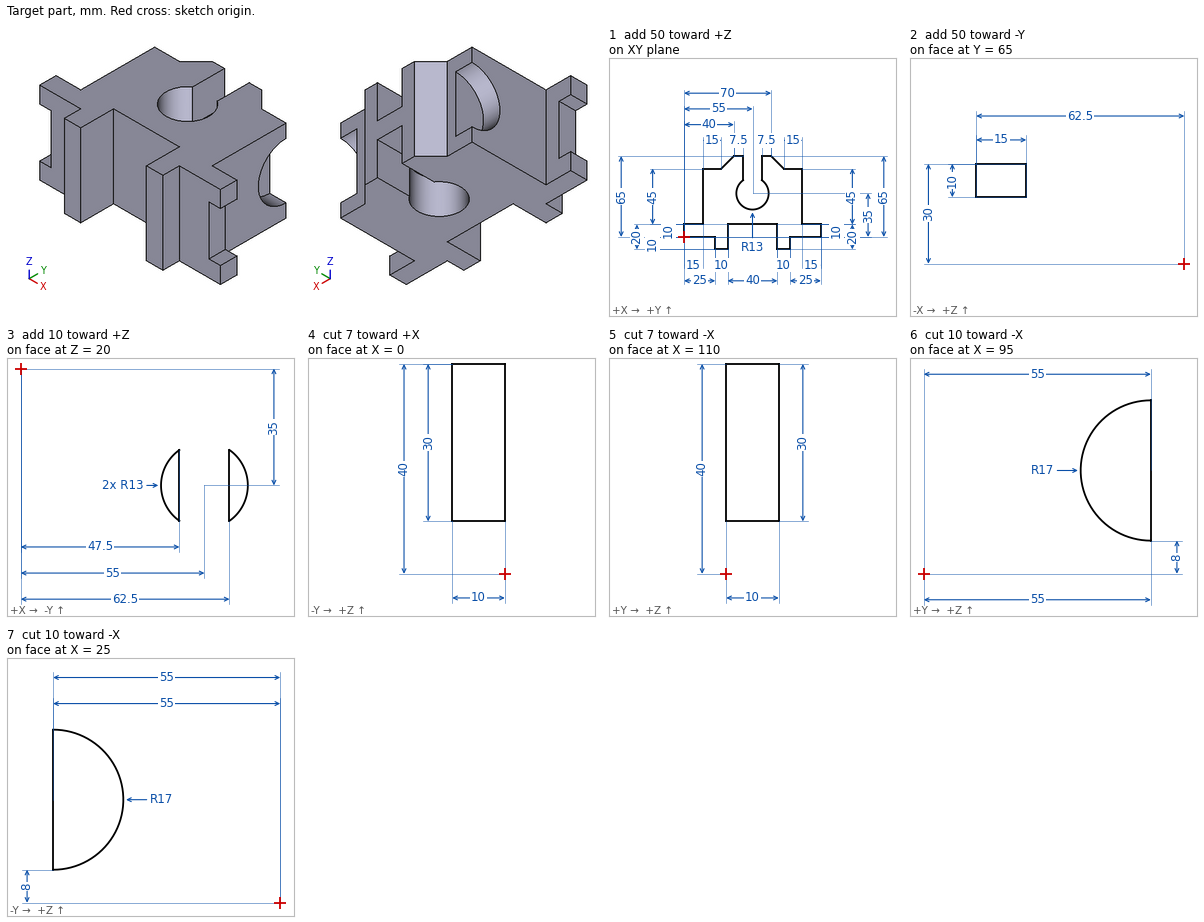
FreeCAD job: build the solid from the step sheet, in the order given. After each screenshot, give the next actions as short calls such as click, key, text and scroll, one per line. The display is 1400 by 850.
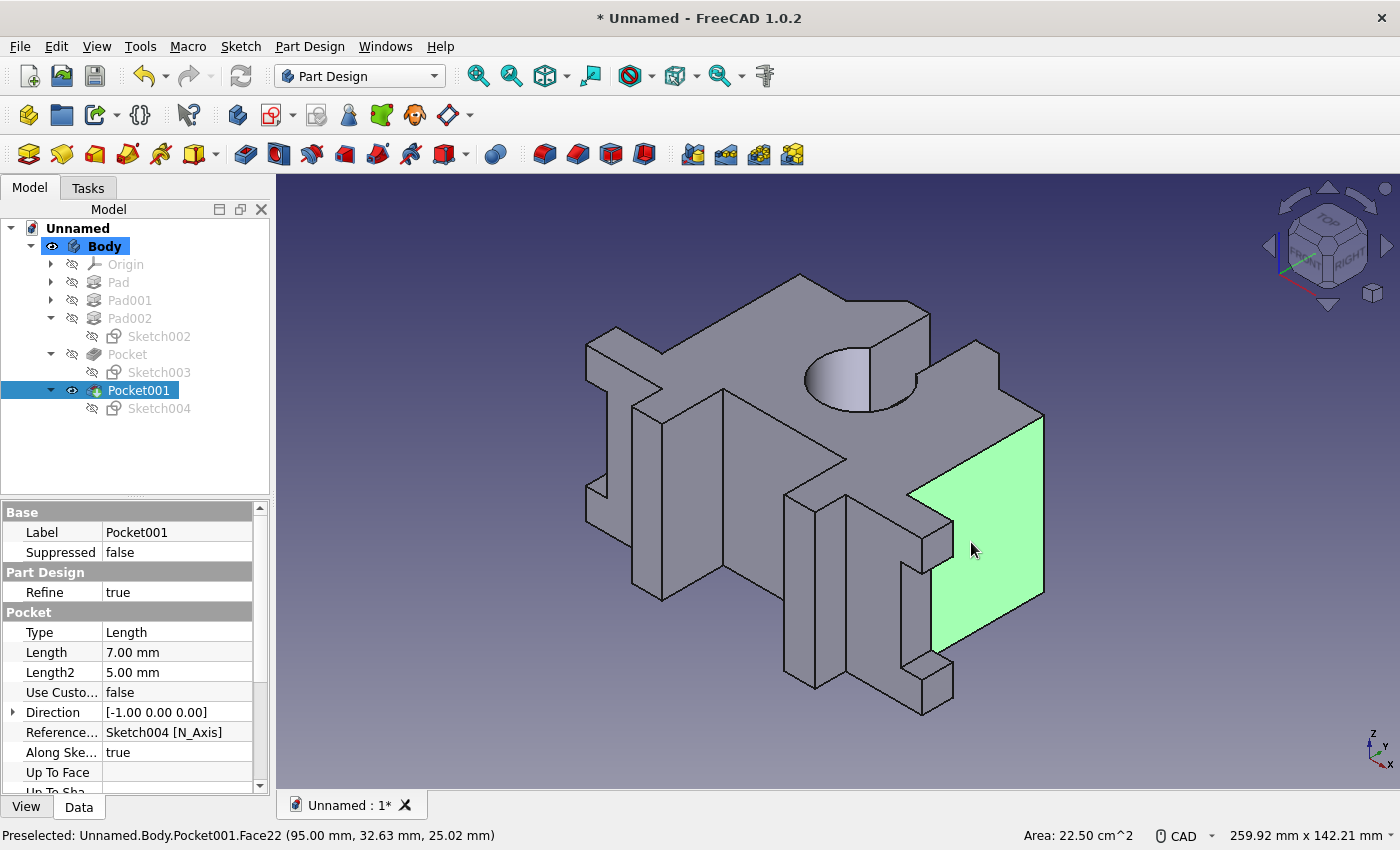
click(270, 116)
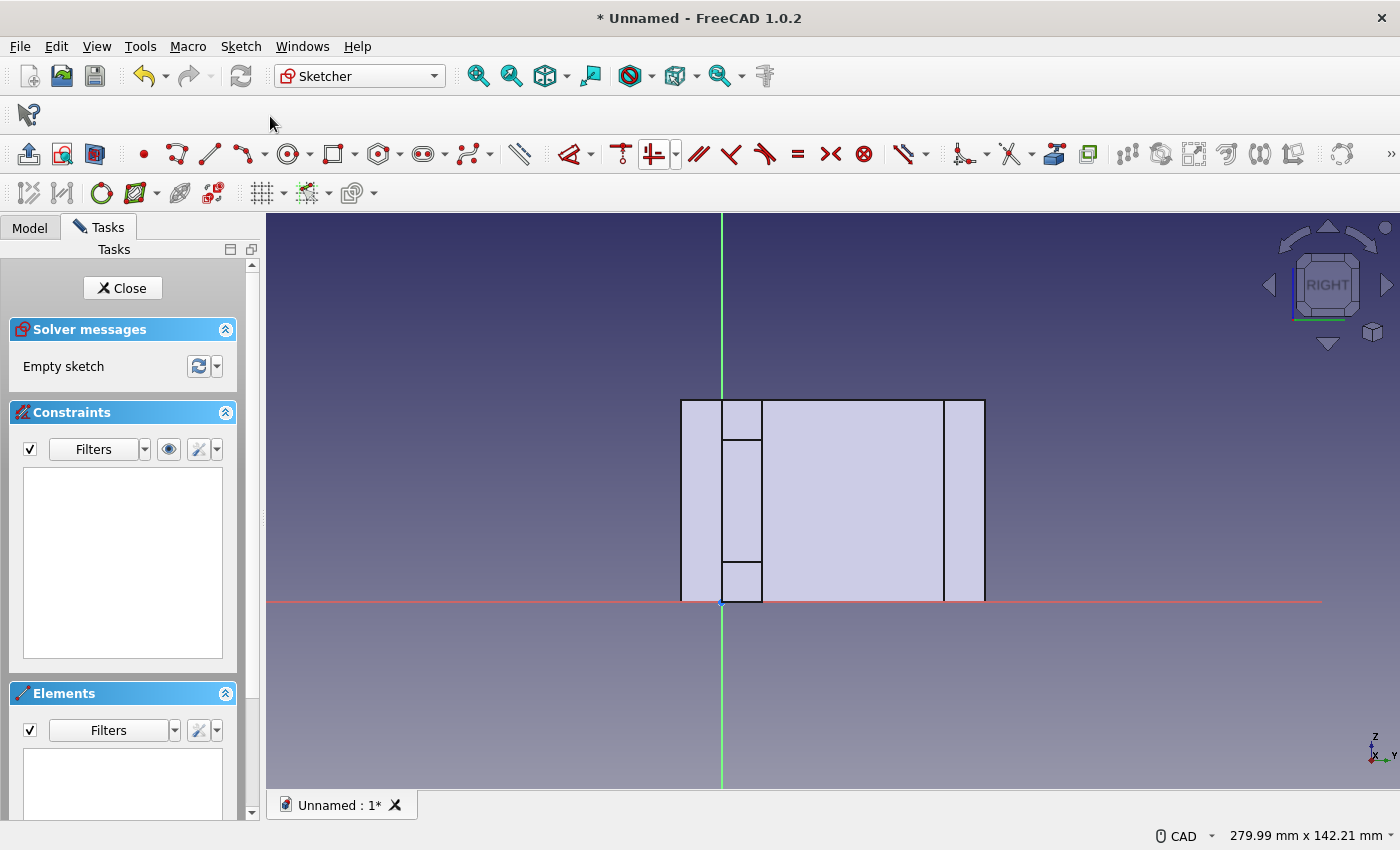
scroll(889, 530, up, 4)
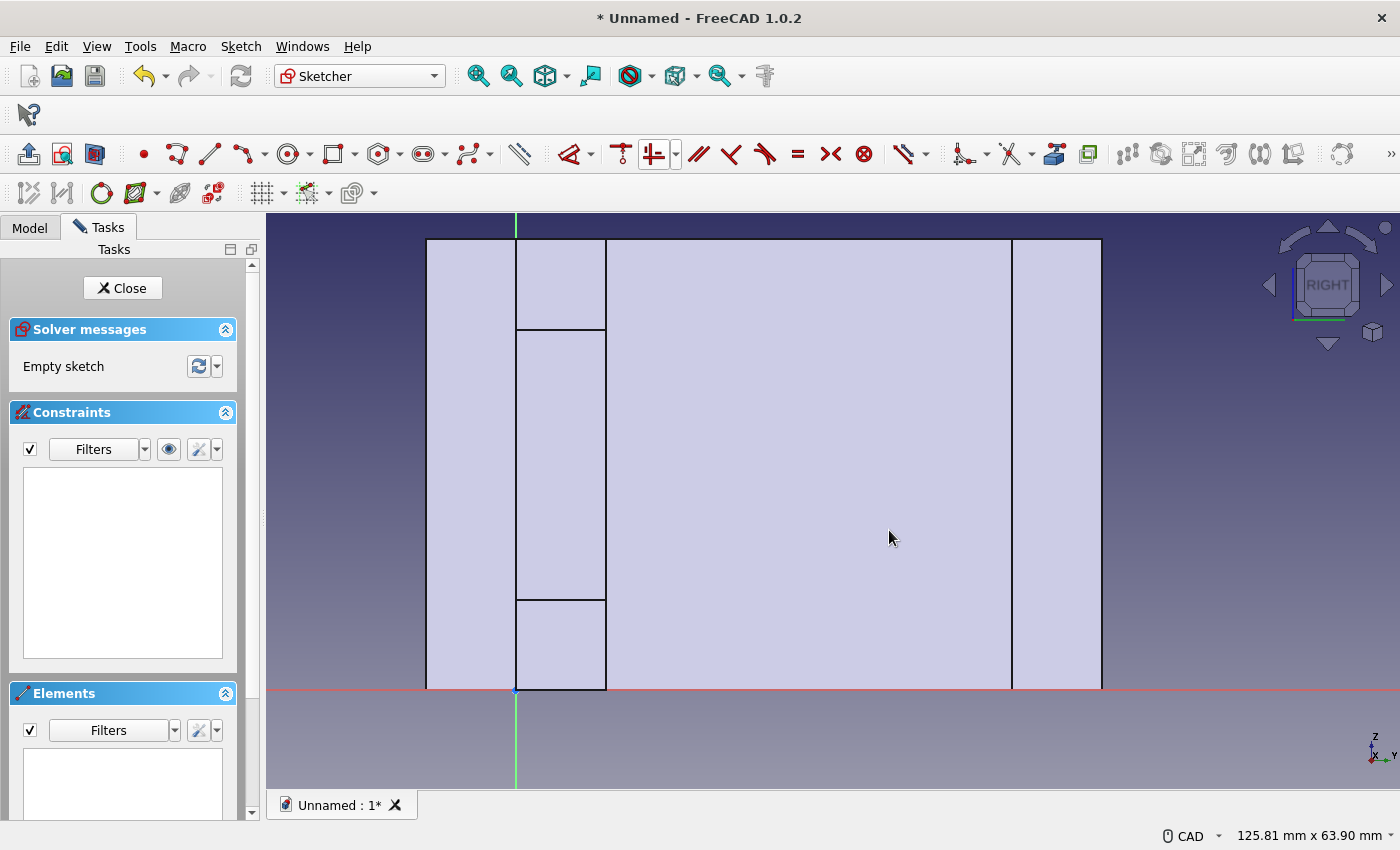
click(210, 154)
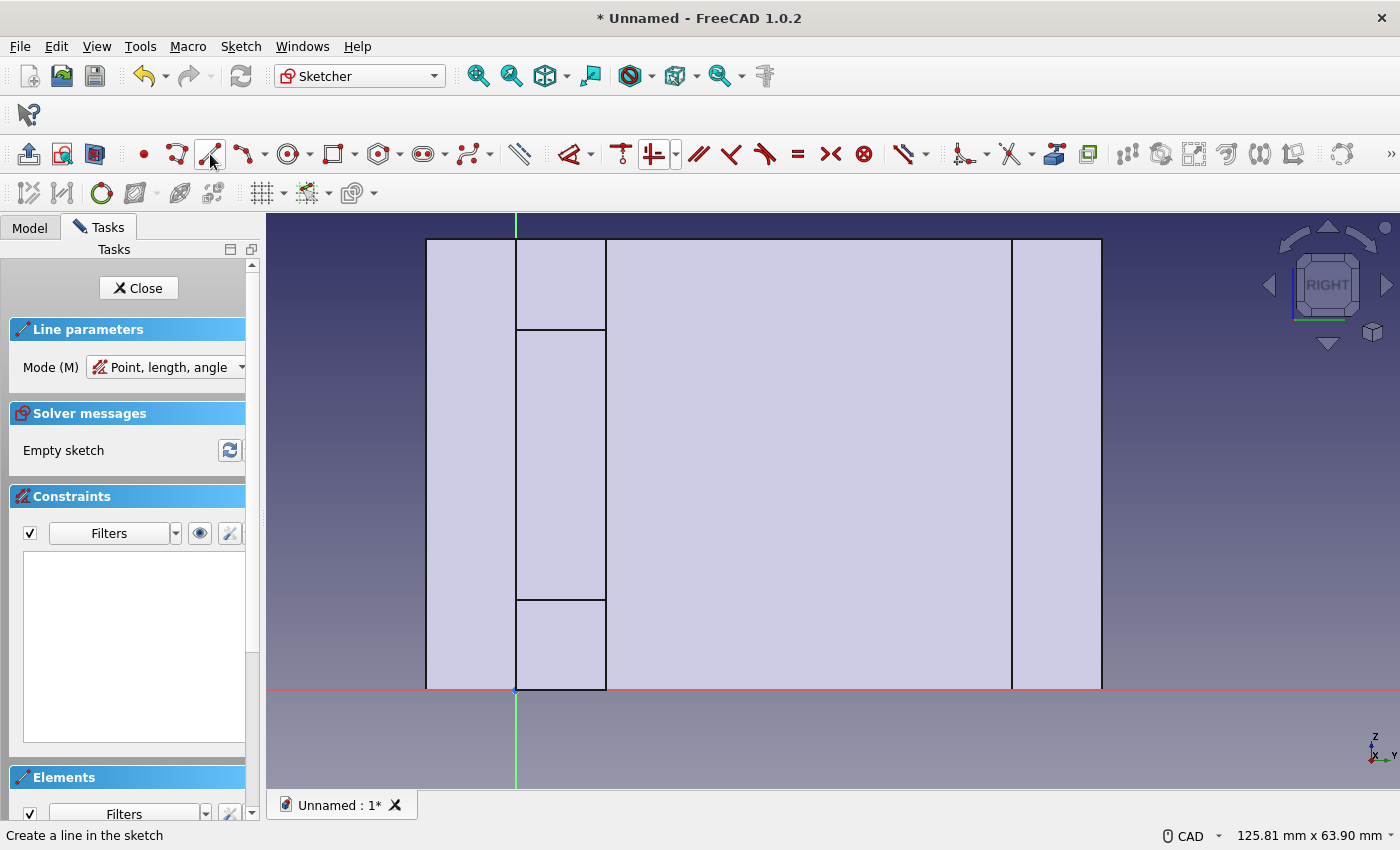
click(1012, 618)
click(1012, 312)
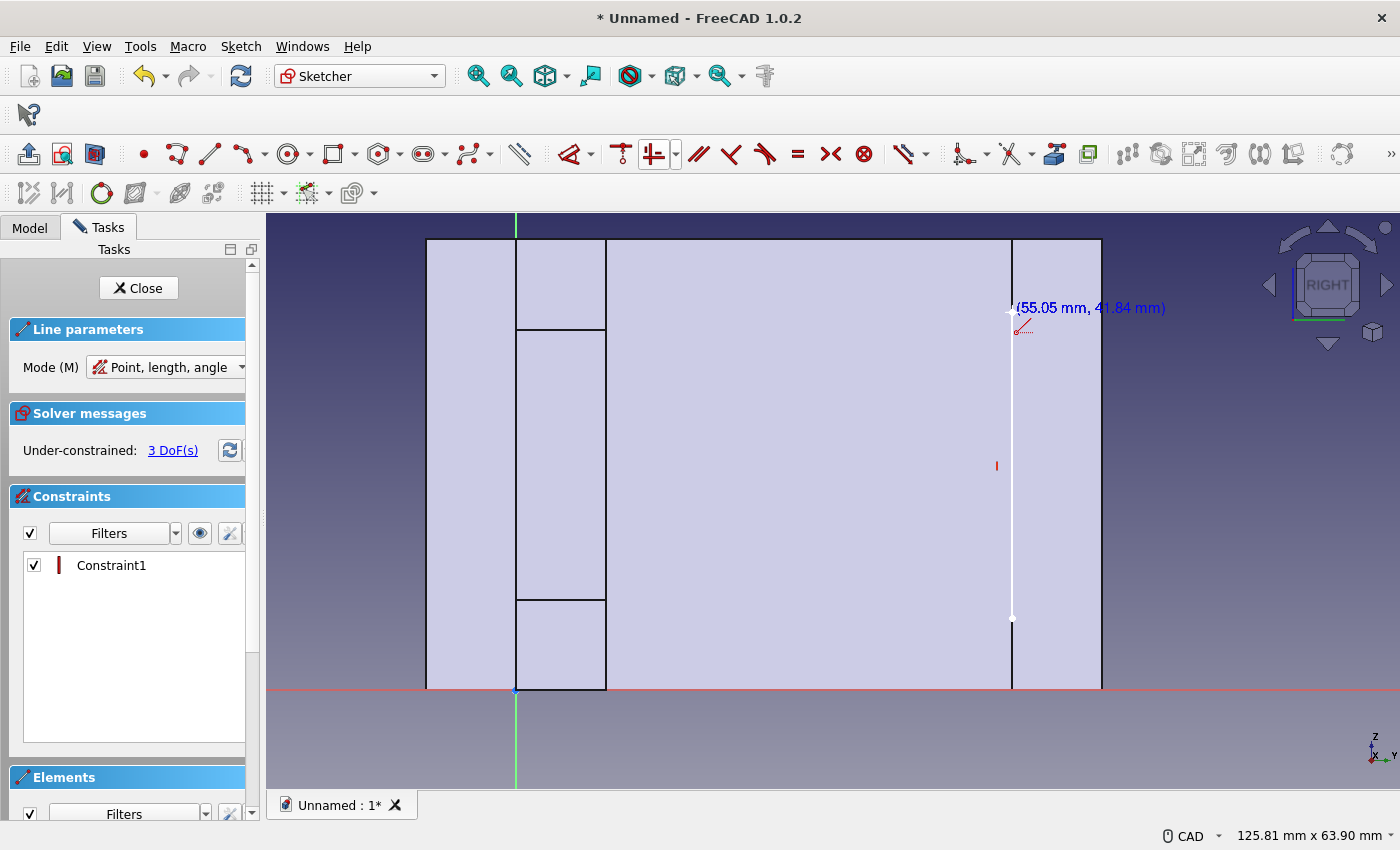
click(242, 154)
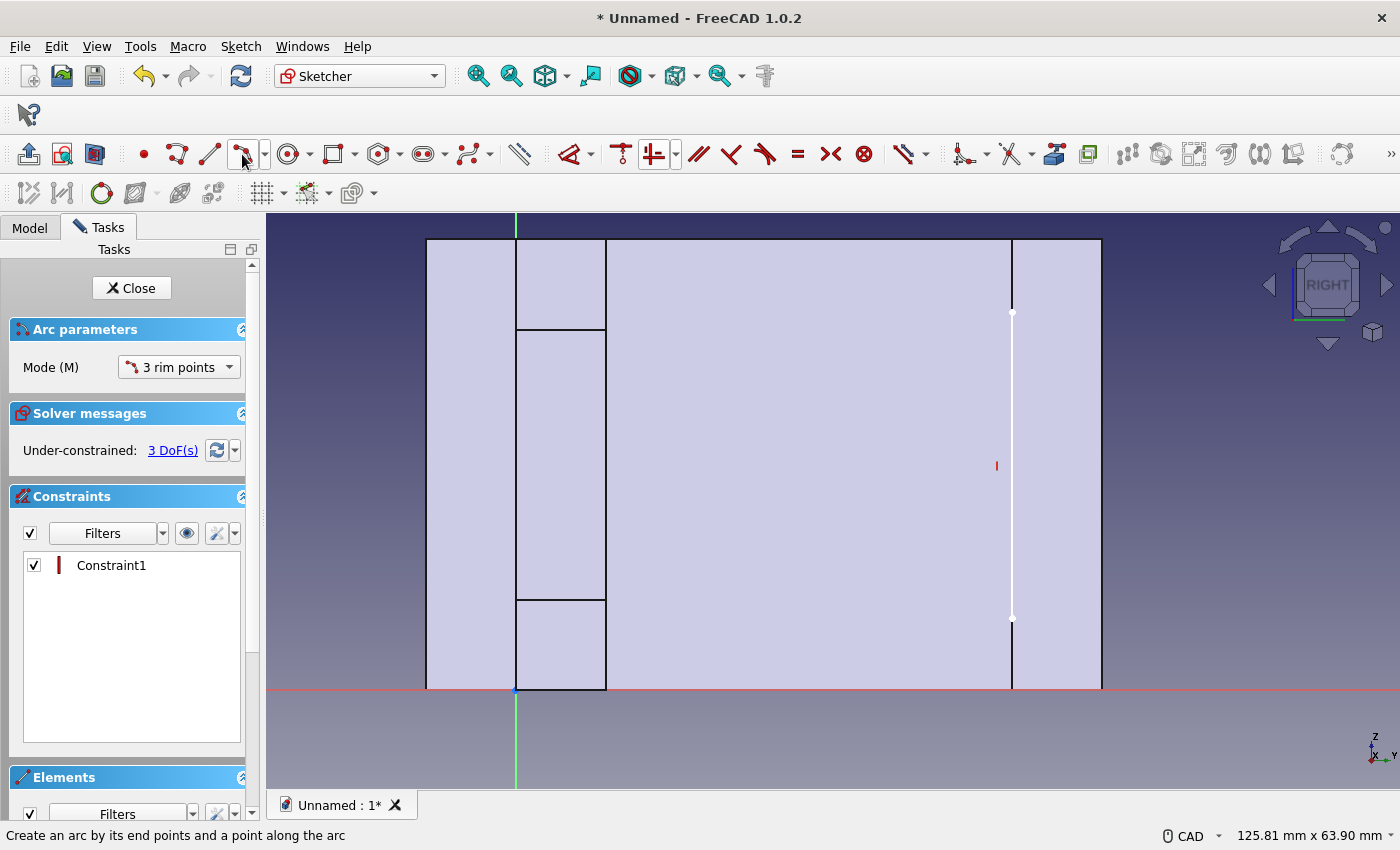
click(1012, 313)
click(1012, 619)
click(858, 465)
key(Escape)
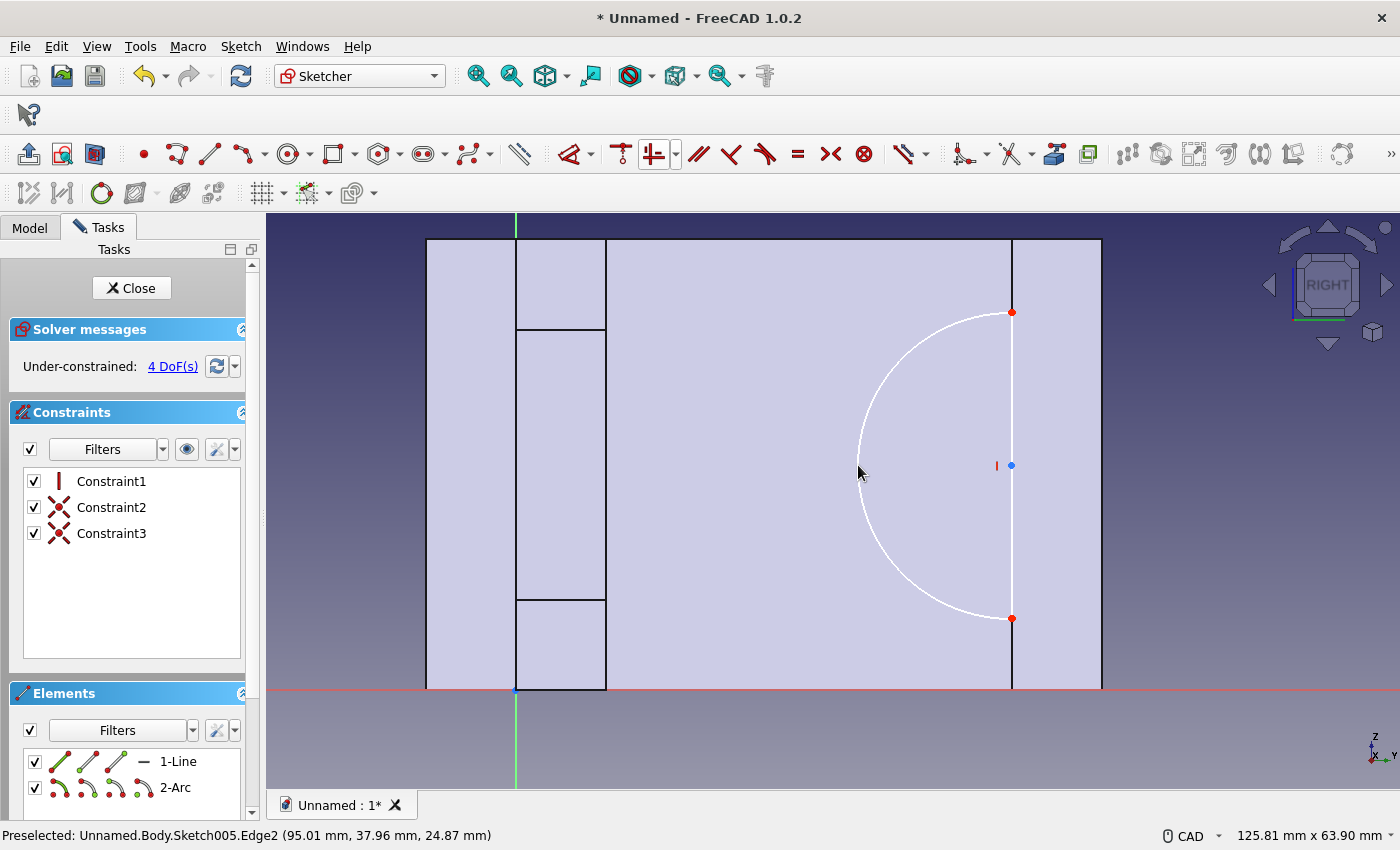
click(568, 154)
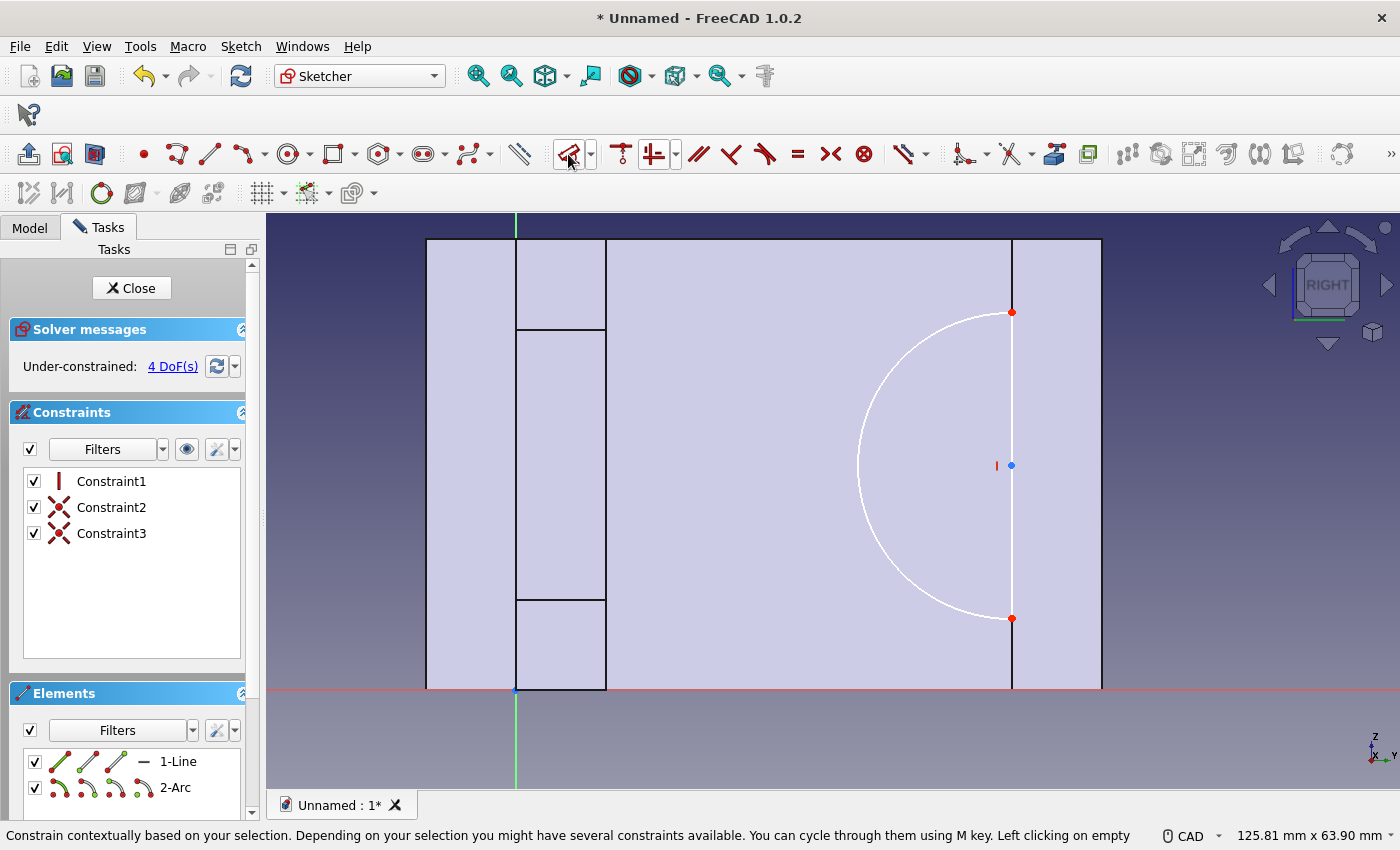
click(887, 376)
click(861, 357)